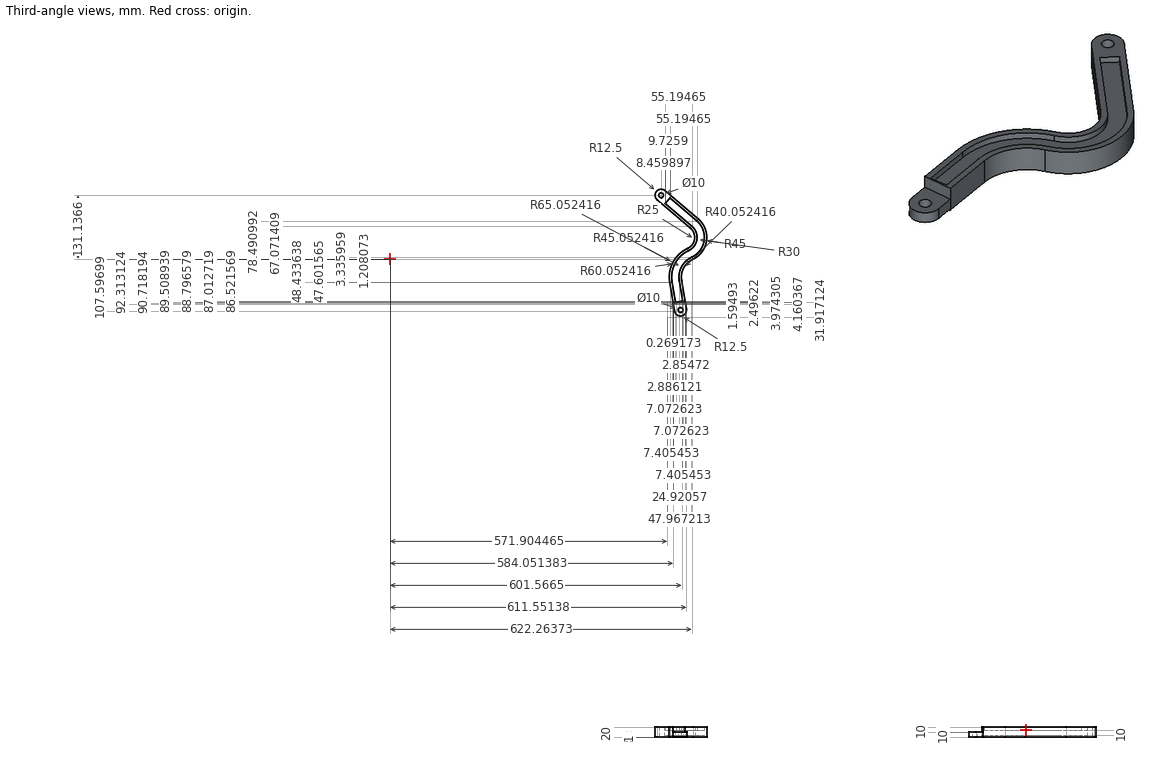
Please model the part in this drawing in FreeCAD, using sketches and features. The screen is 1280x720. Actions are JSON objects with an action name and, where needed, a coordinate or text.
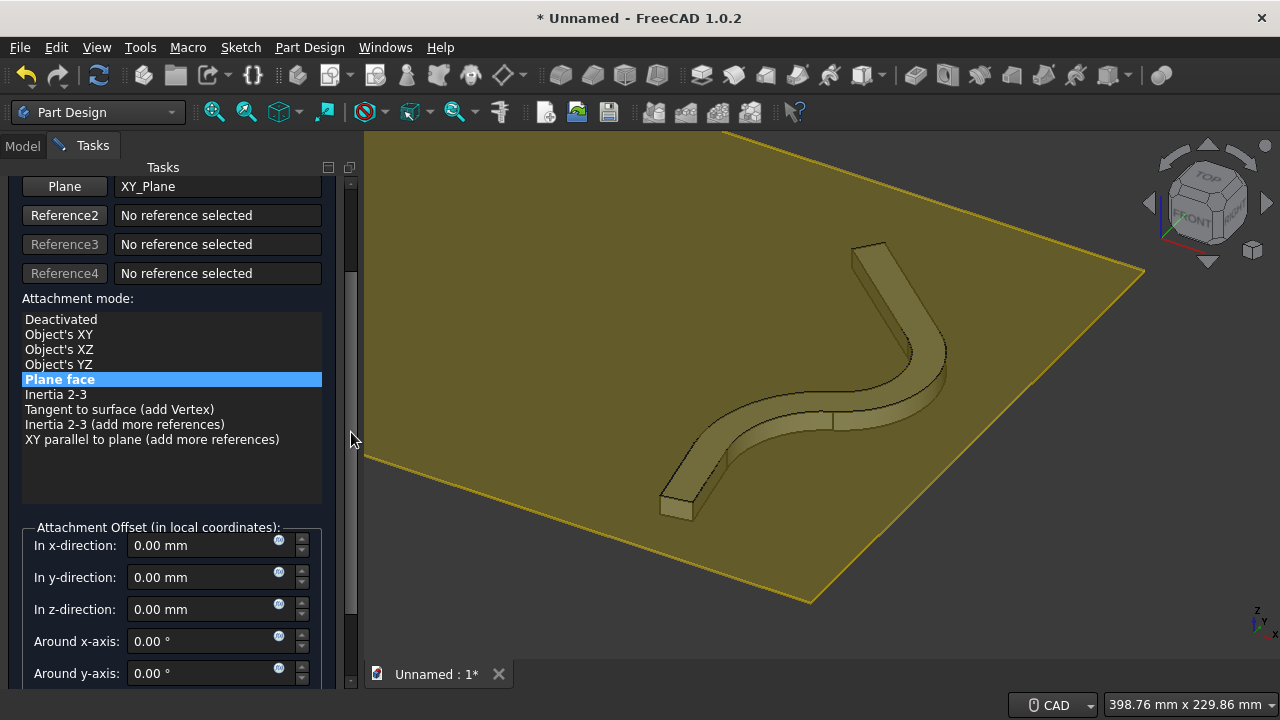
{"action": "triple_click", "coordinate": [210, 609]}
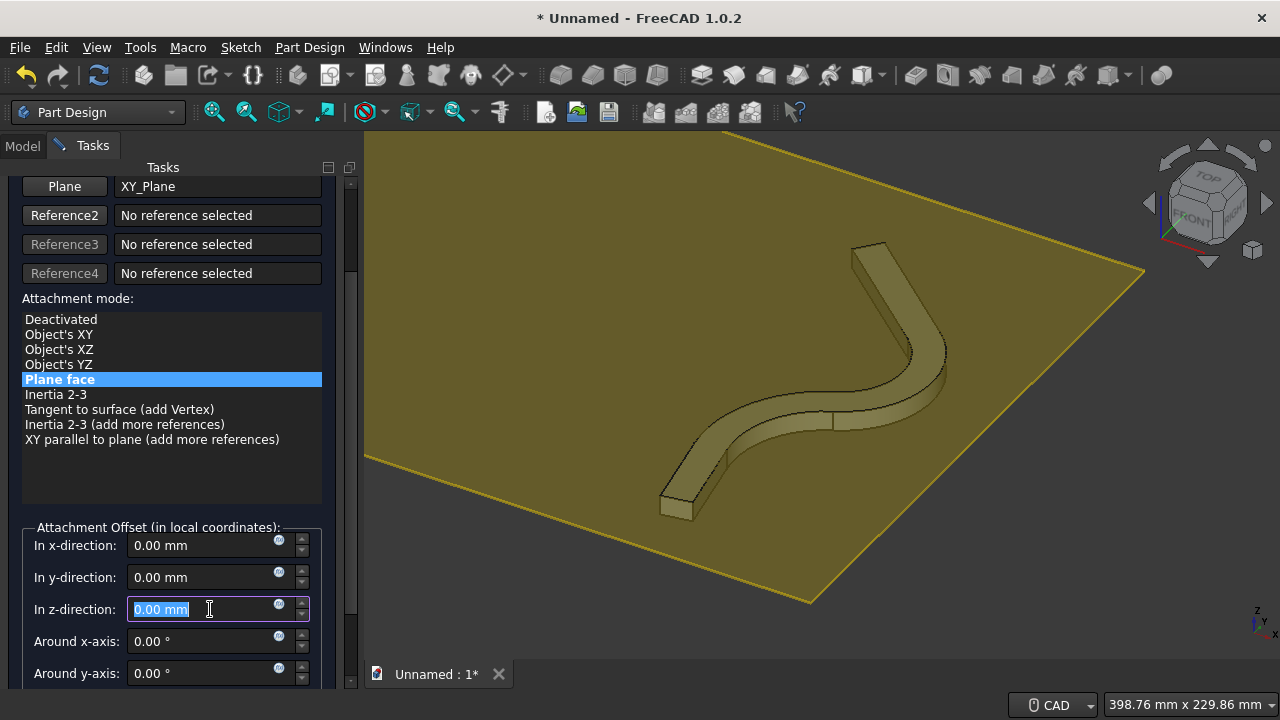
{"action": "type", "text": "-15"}
{"action": "key", "text": "Tab"}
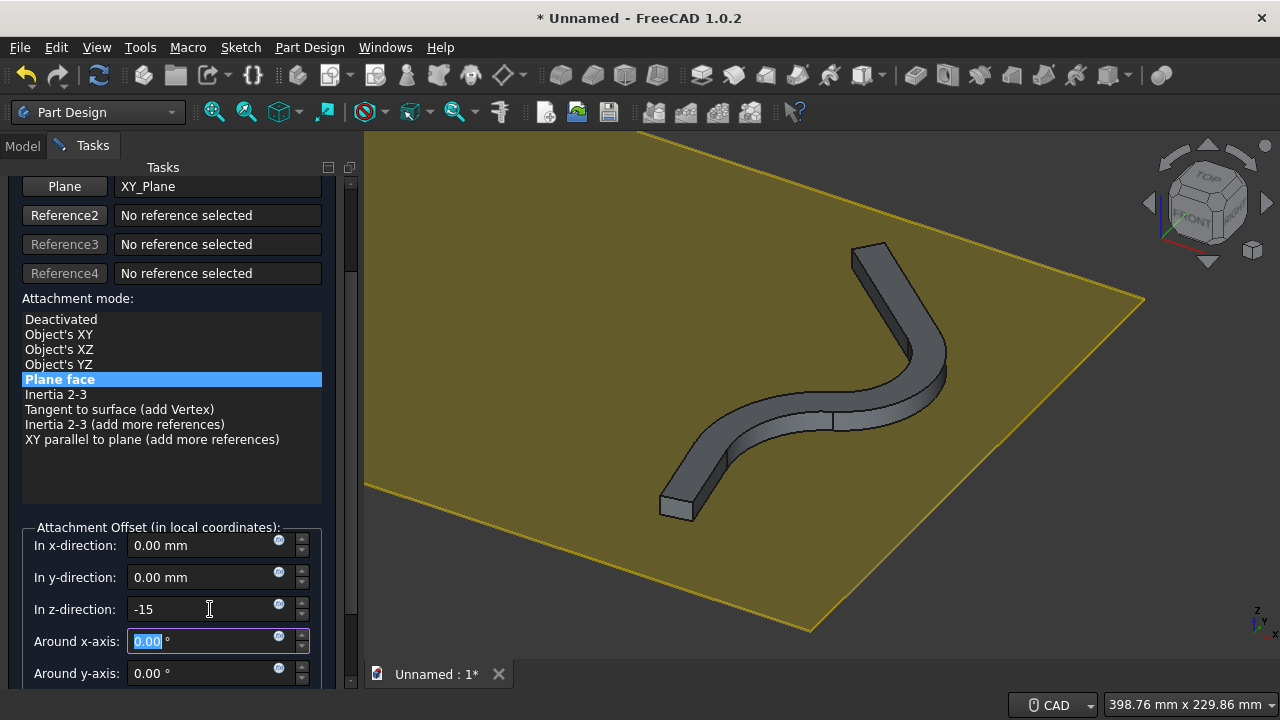
{"action": "scroll", "coordinate": [351, 432], "scroll_direction": "up", "scroll_amount": 3}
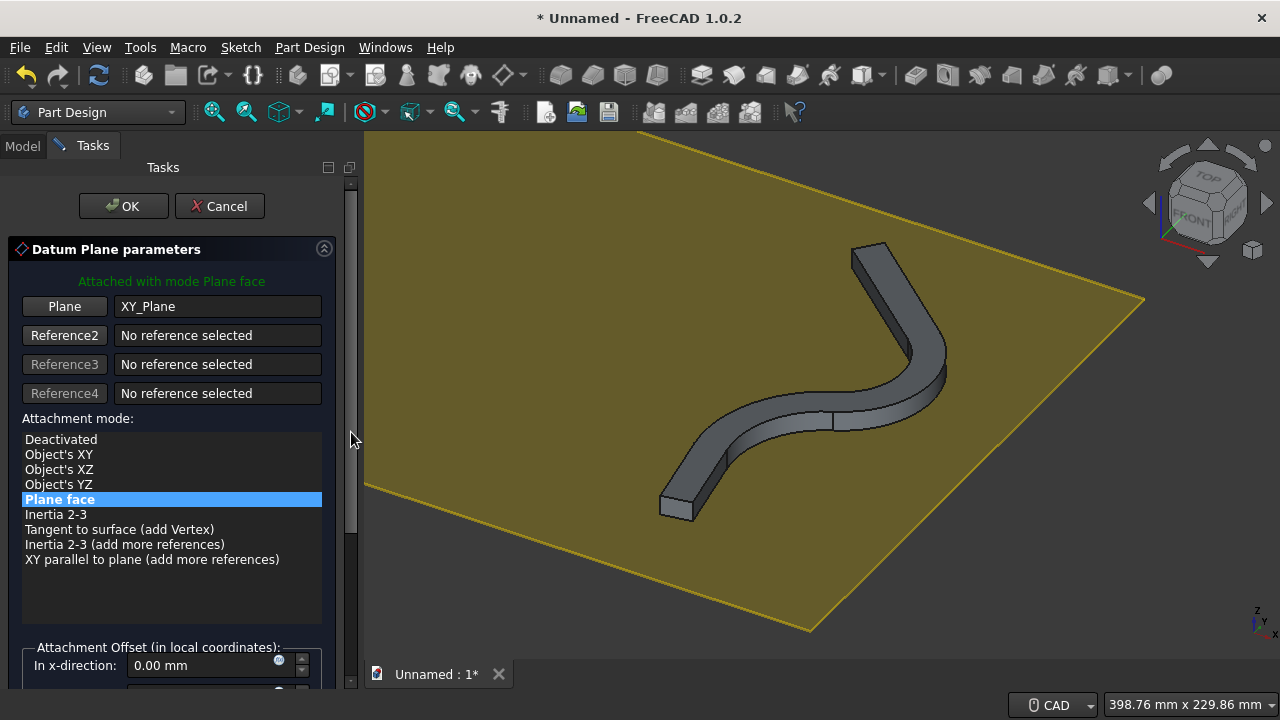
{"action": "left_click", "coordinate": [124, 206]}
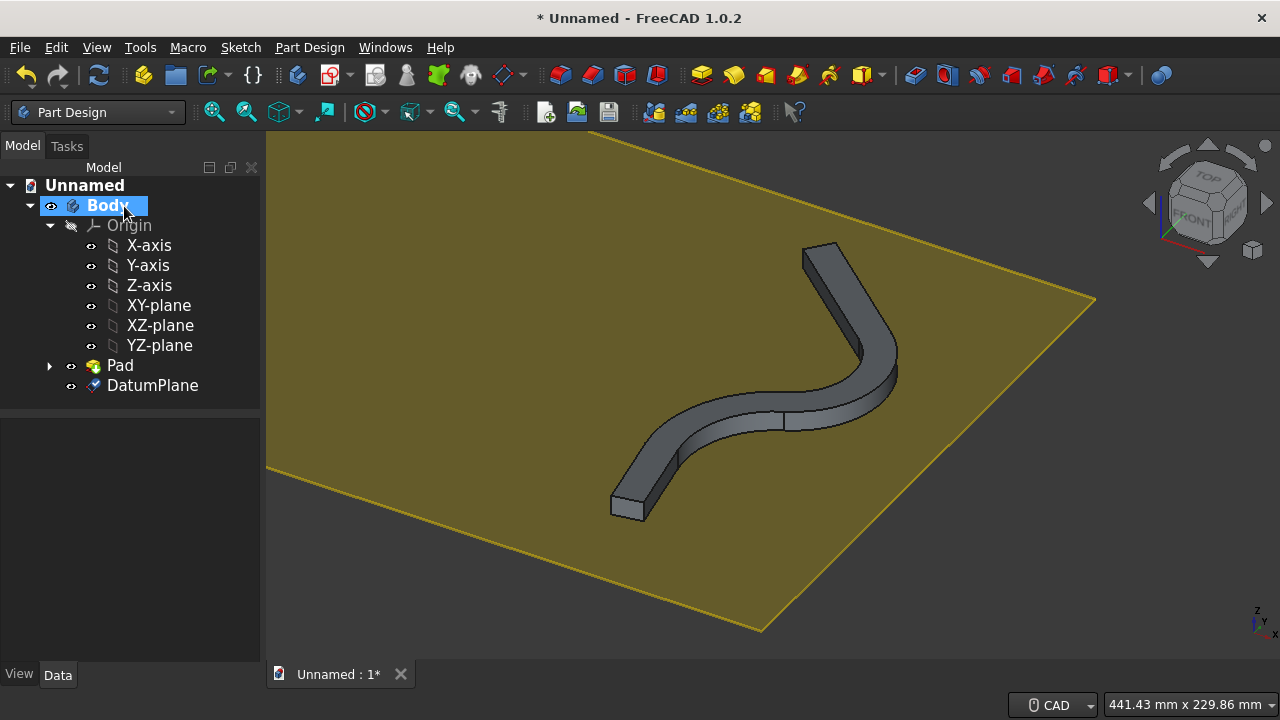
{"action": "left_click", "coordinate": [116, 386]}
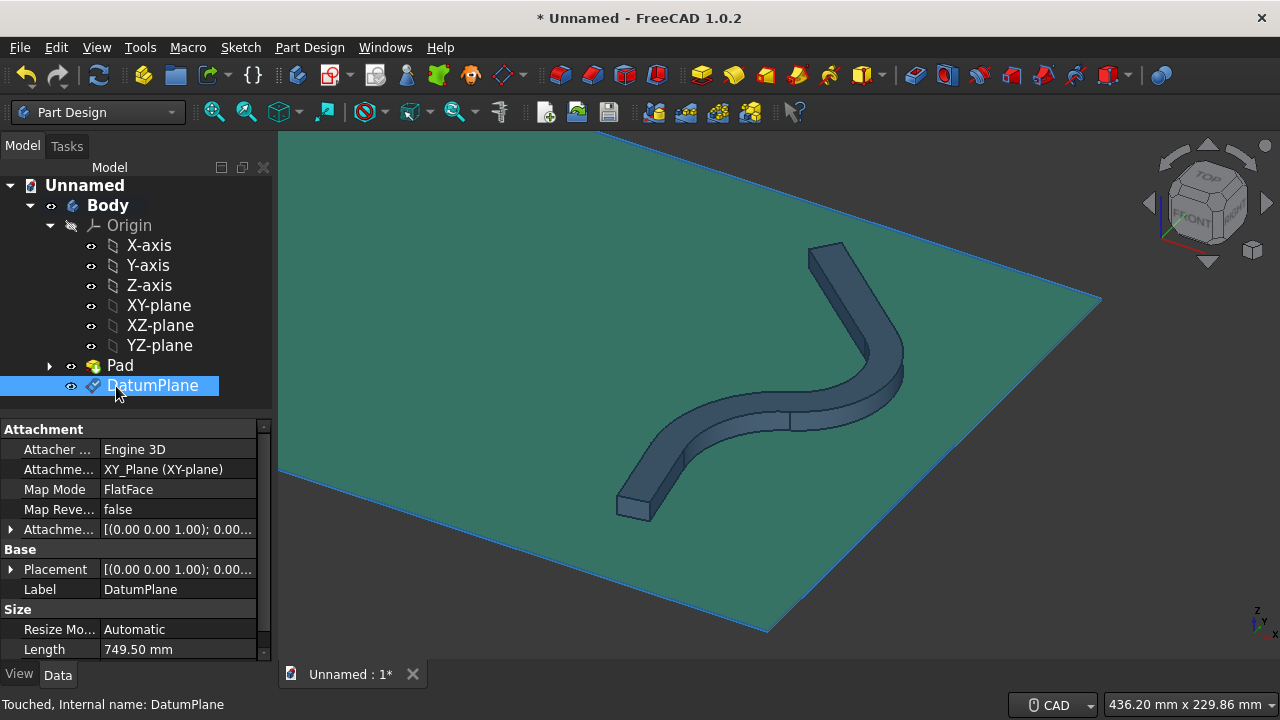
{"action": "left_click", "coordinate": [330, 76]}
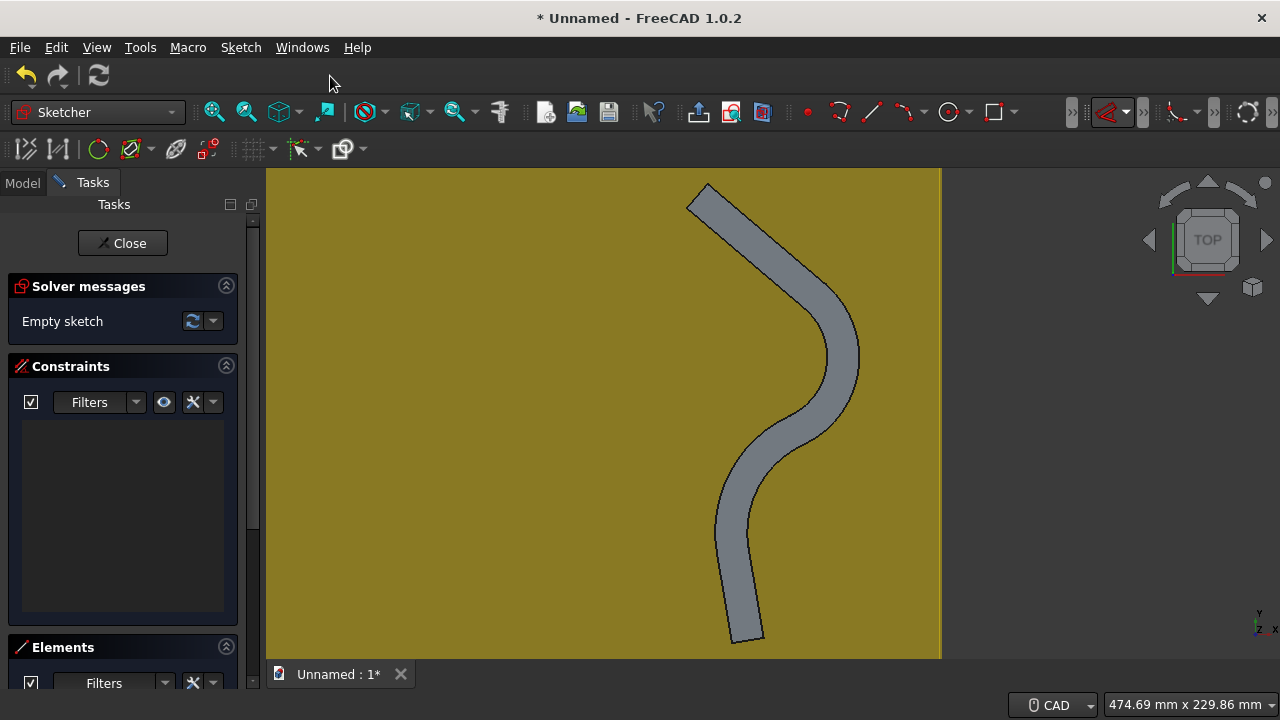
{"action": "key", "text": "q s"}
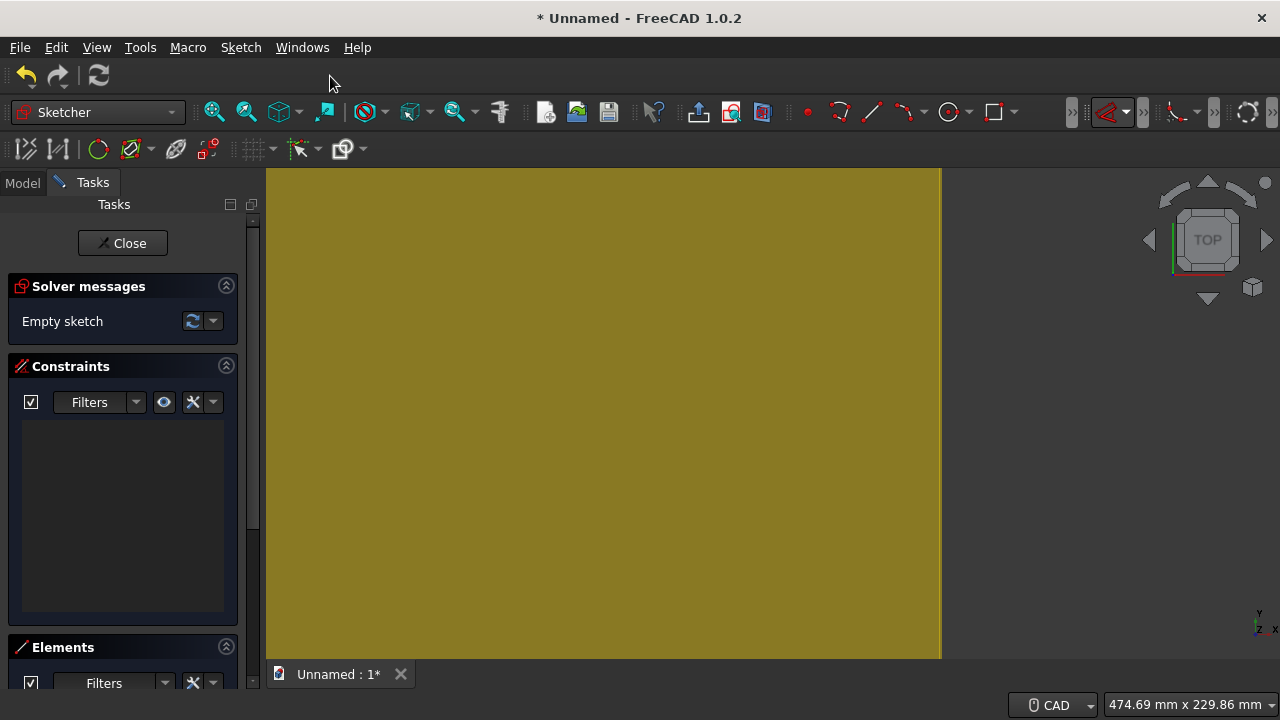
{"action": "scroll", "coordinate": [594, 440], "scroll_direction": "down", "scroll_amount": 2}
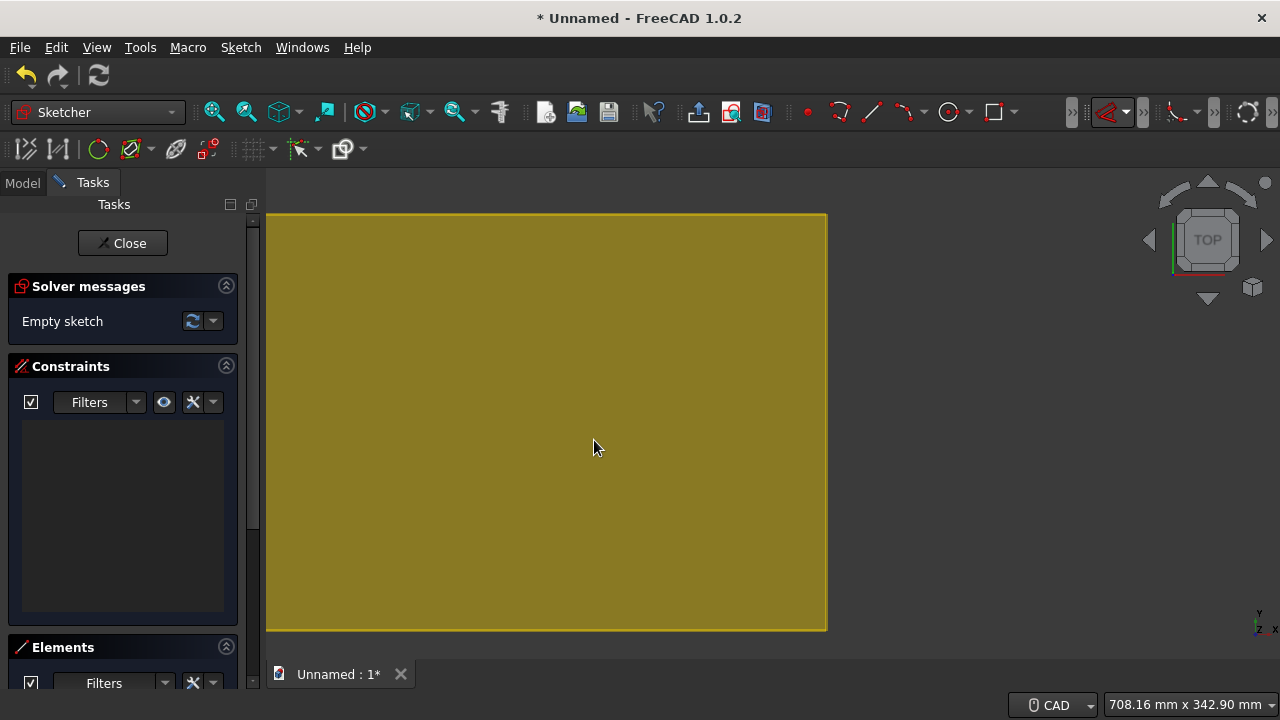
{"action": "left_click", "coordinate": [872, 112]}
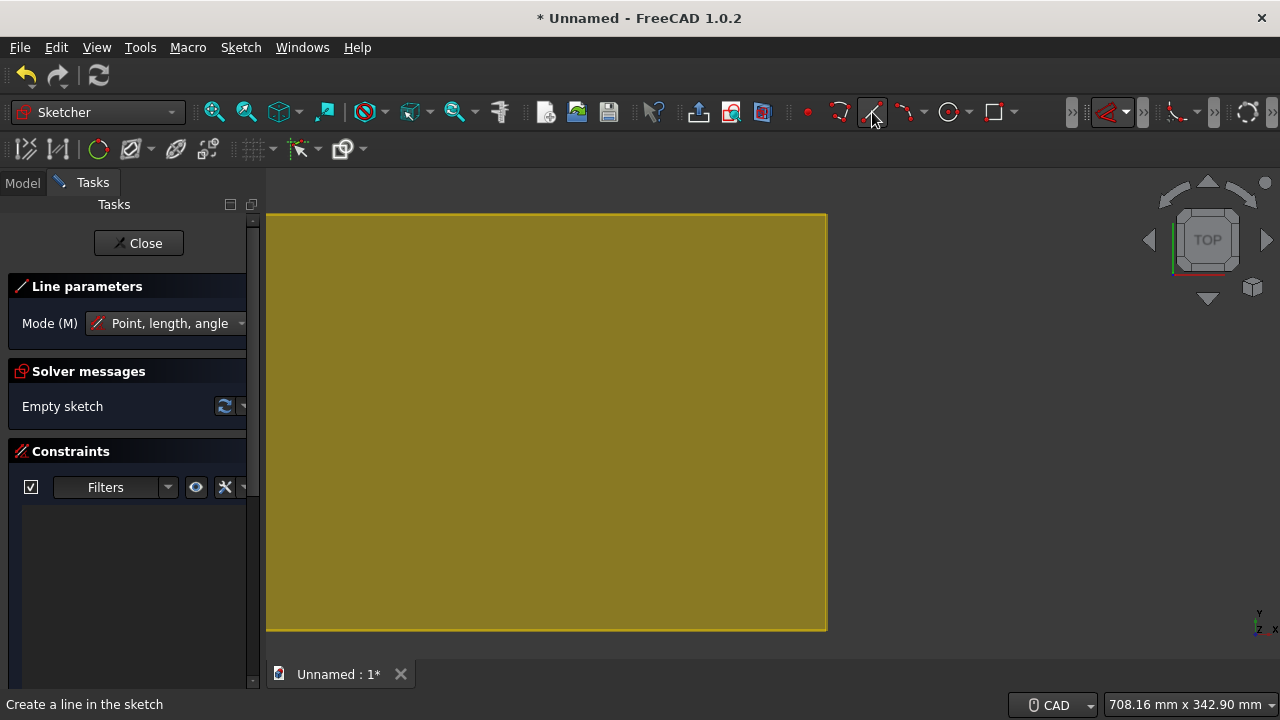
{"action": "left_click", "coordinate": [754, 330]}
{"action": "left_click", "coordinate": [656, 247]}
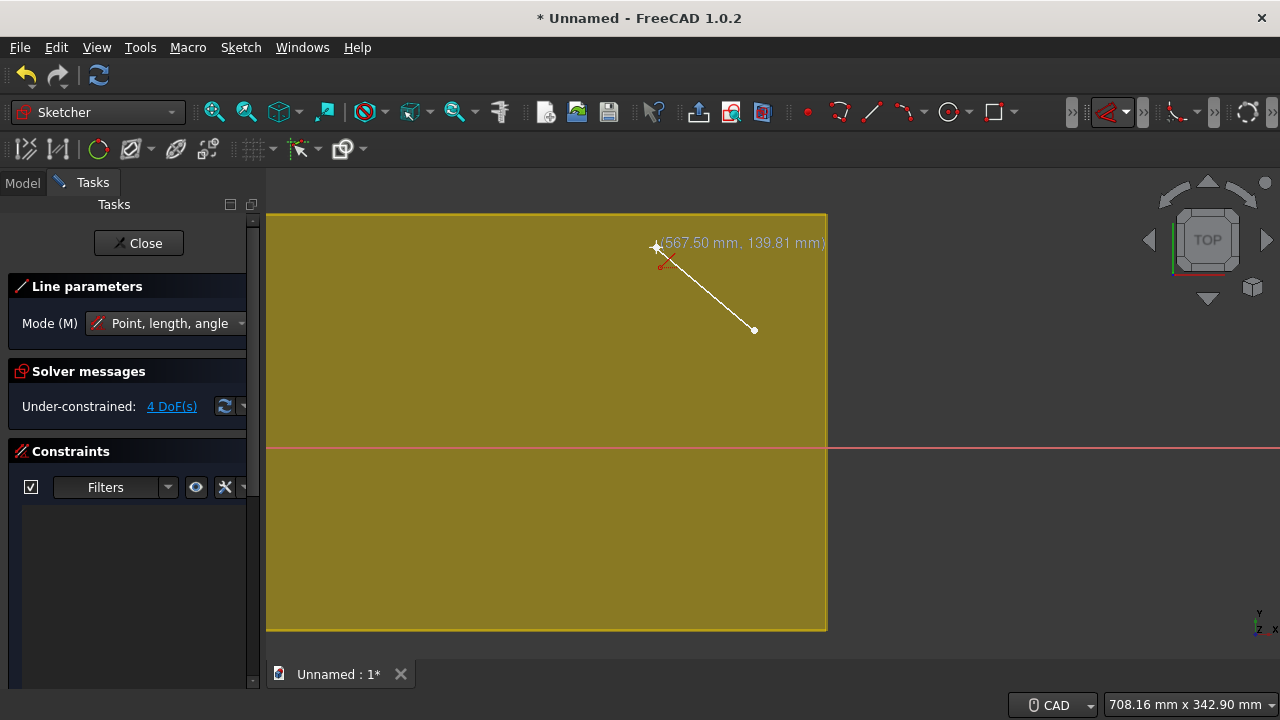
{"action": "left_click", "coordinate": [633, 274]}
{"action": "left_click", "coordinate": [731, 358]}